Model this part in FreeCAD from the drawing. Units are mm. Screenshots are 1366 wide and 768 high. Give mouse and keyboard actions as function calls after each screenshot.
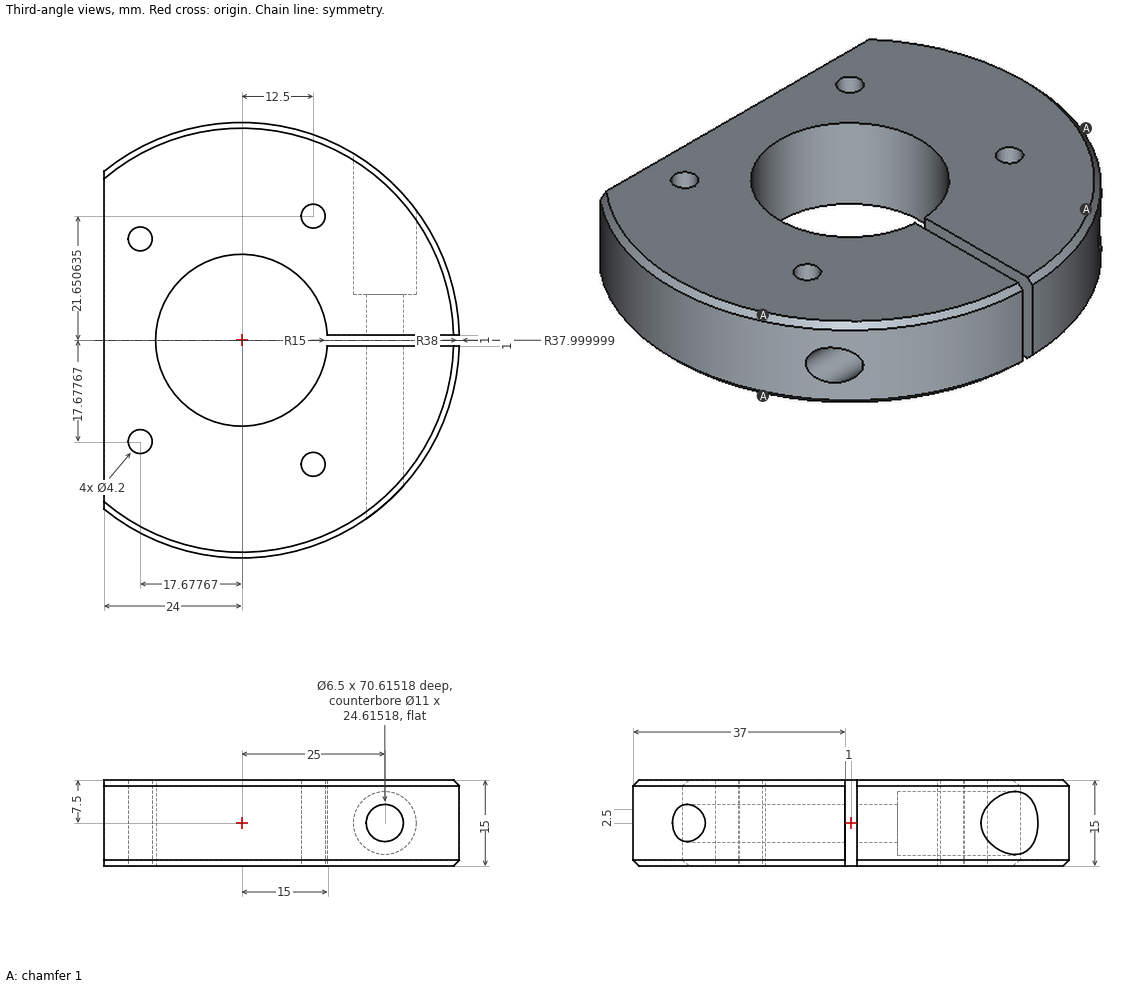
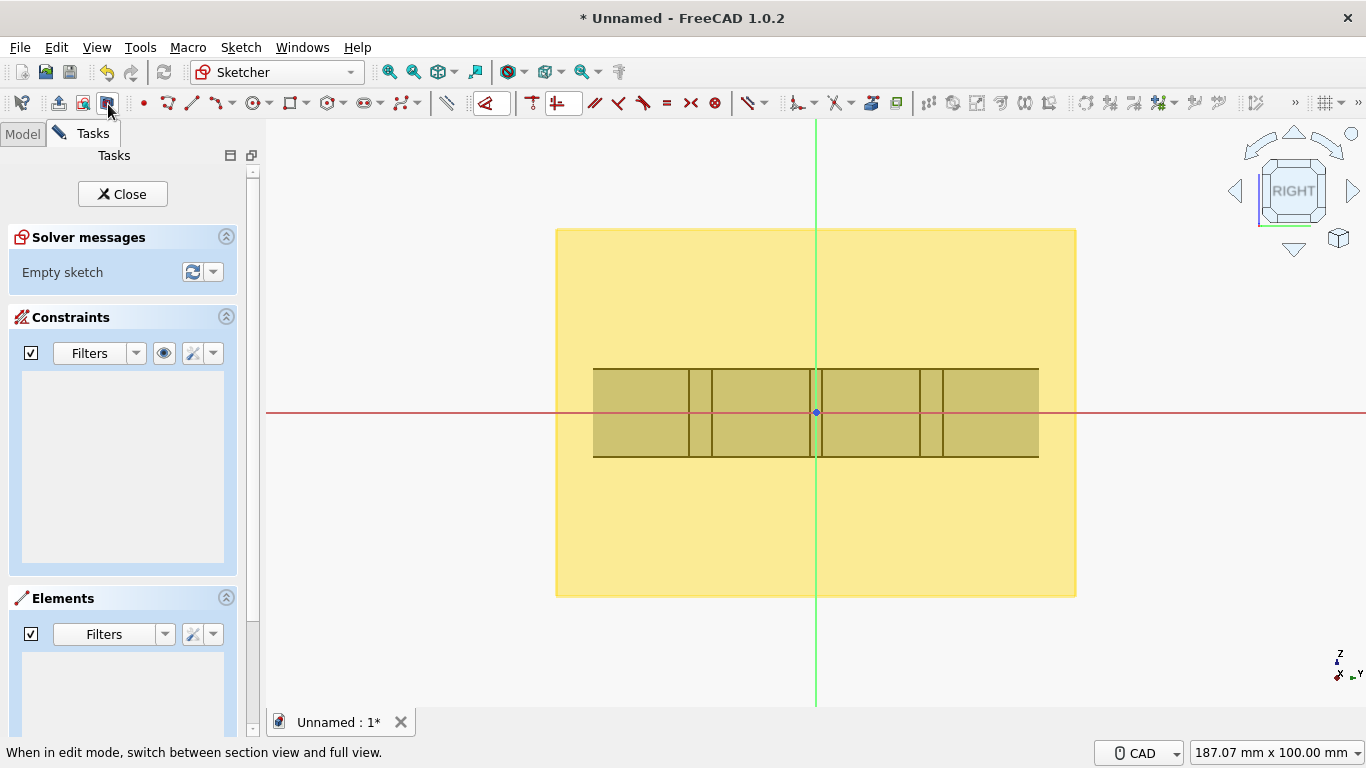
scroll(679, 401, up, 5)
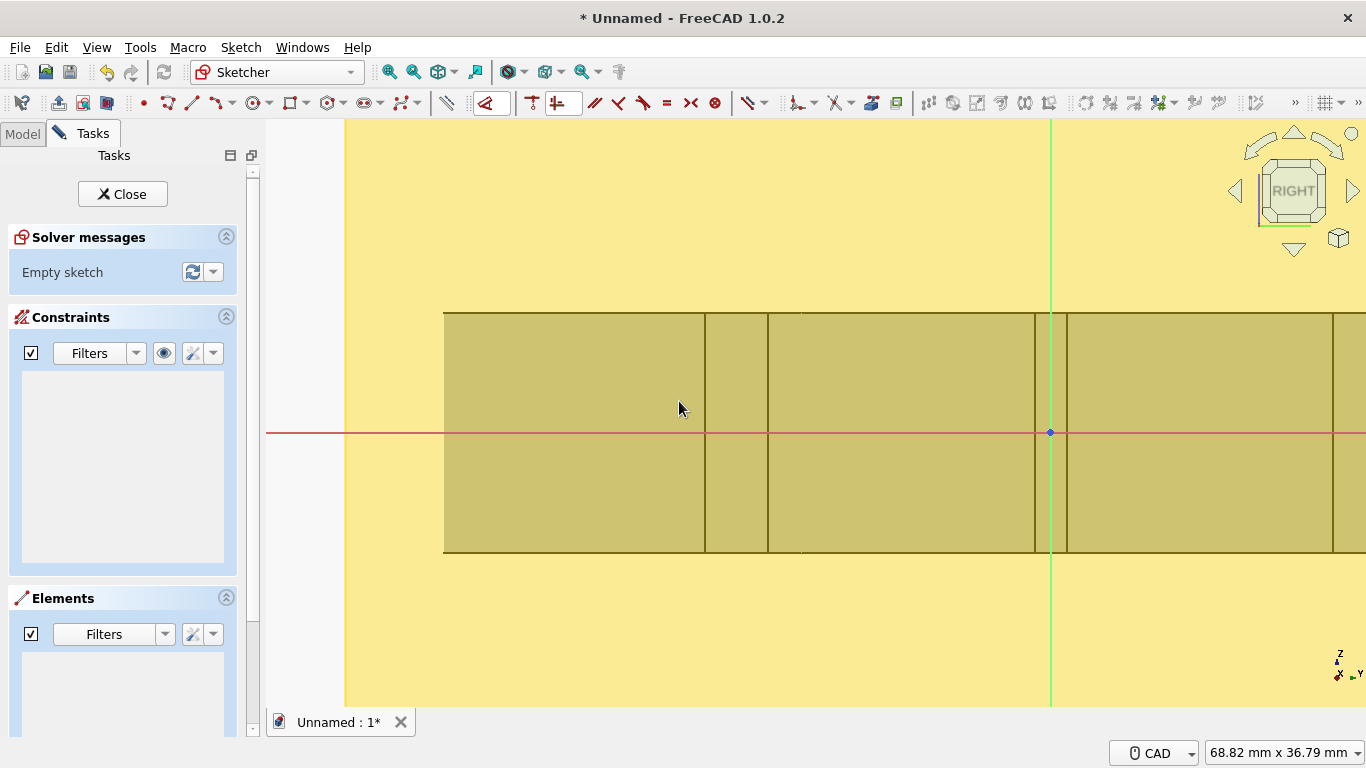
click(290, 104)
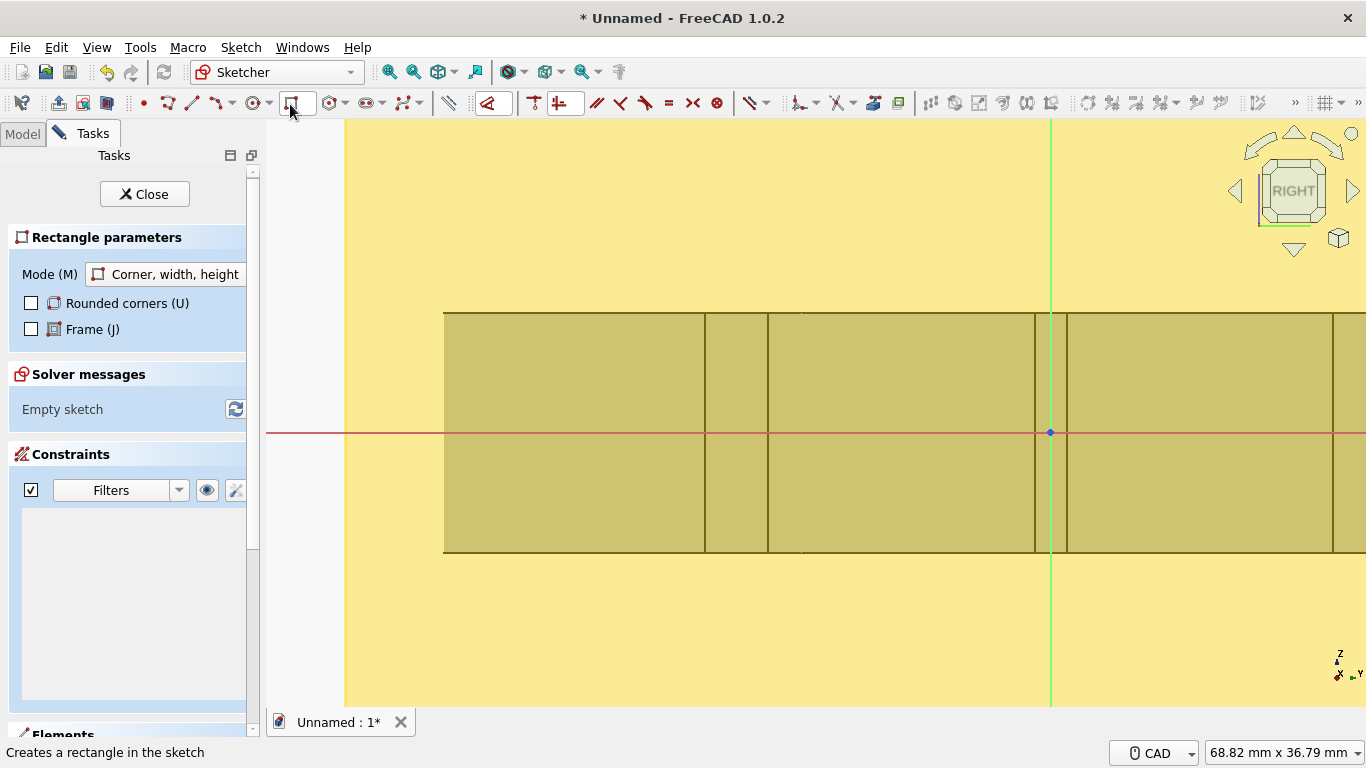
click(443, 393)
click(1035, 433)
key(Escape)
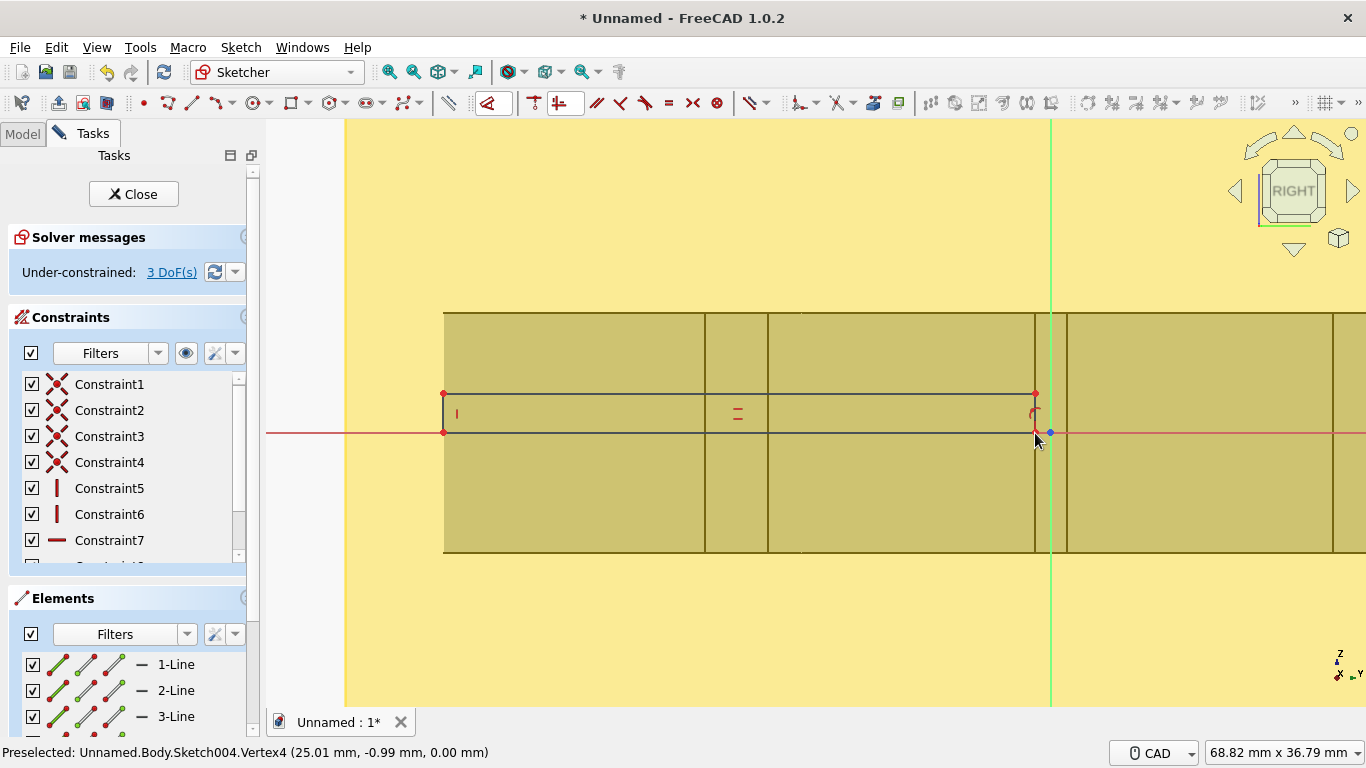
click(621, 433)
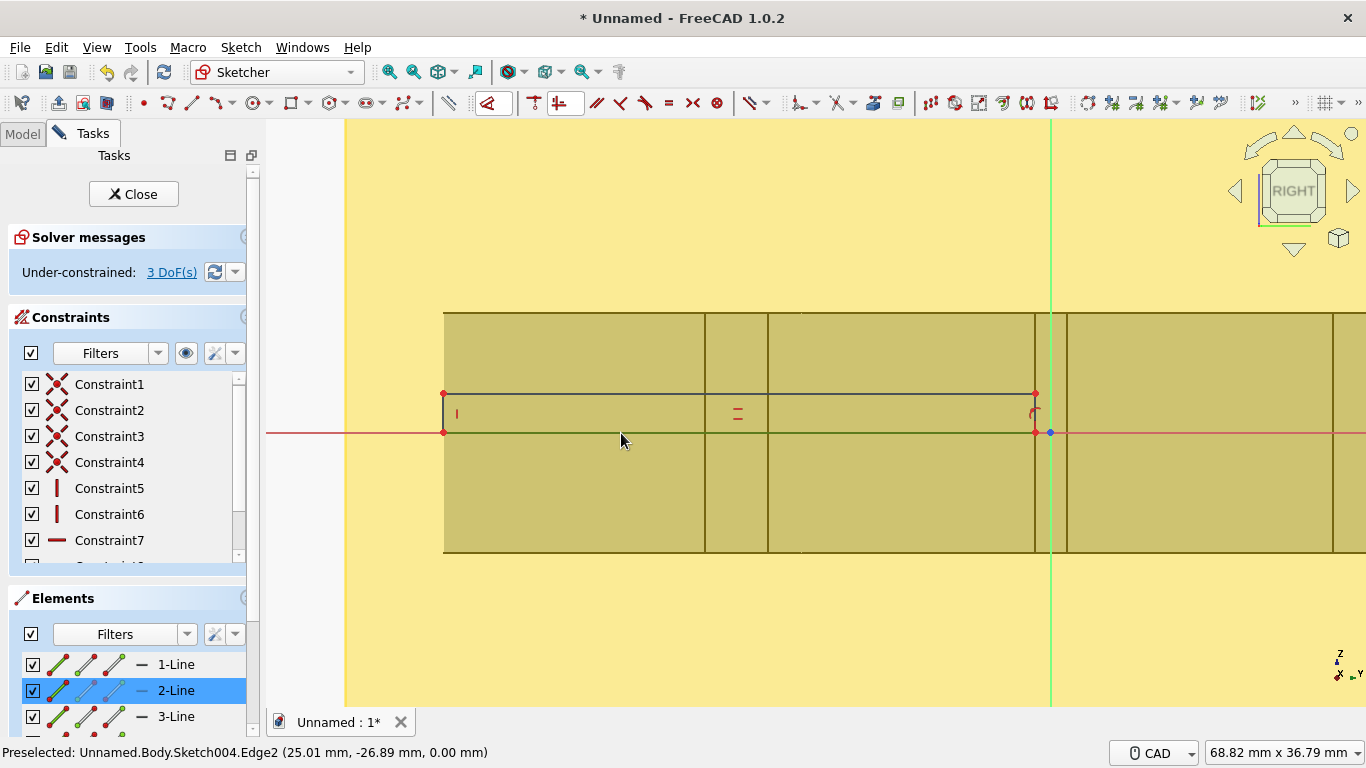
key(l)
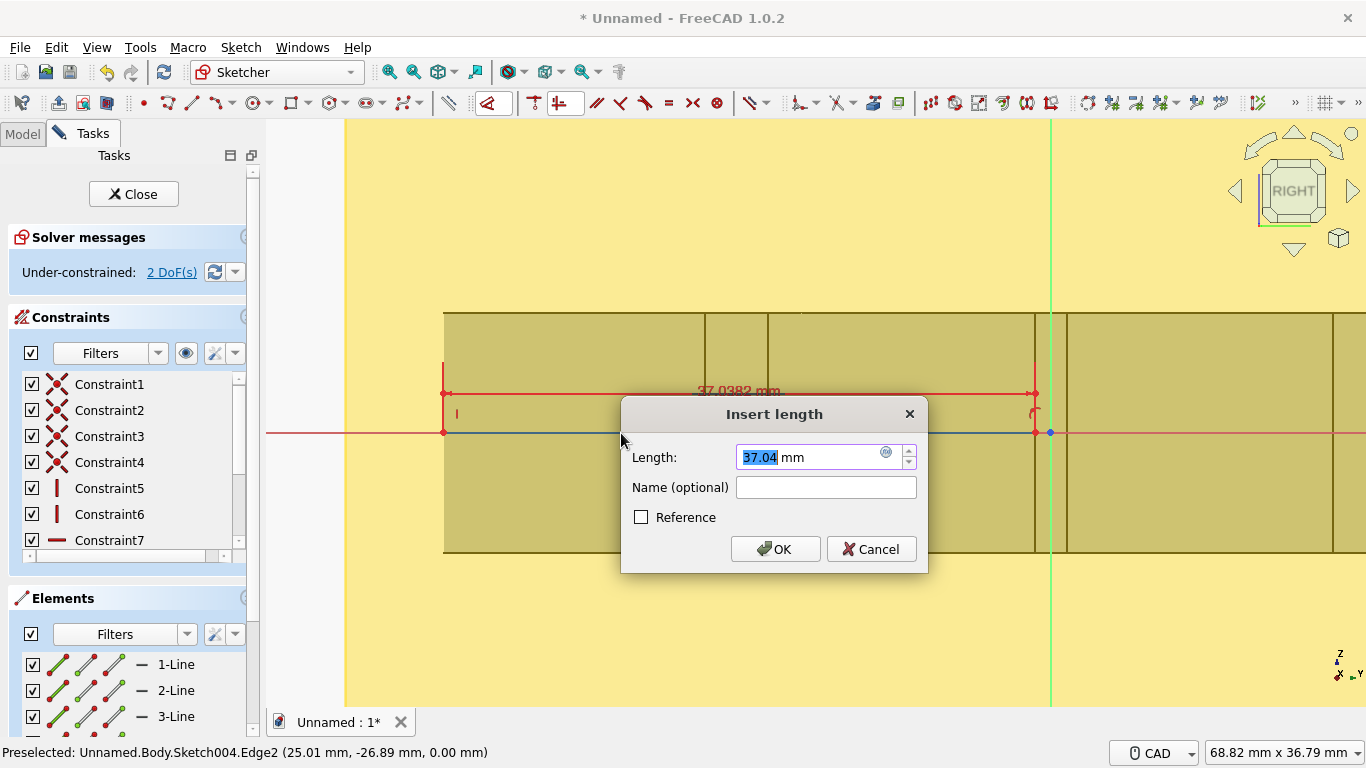
text(37)
key(Return)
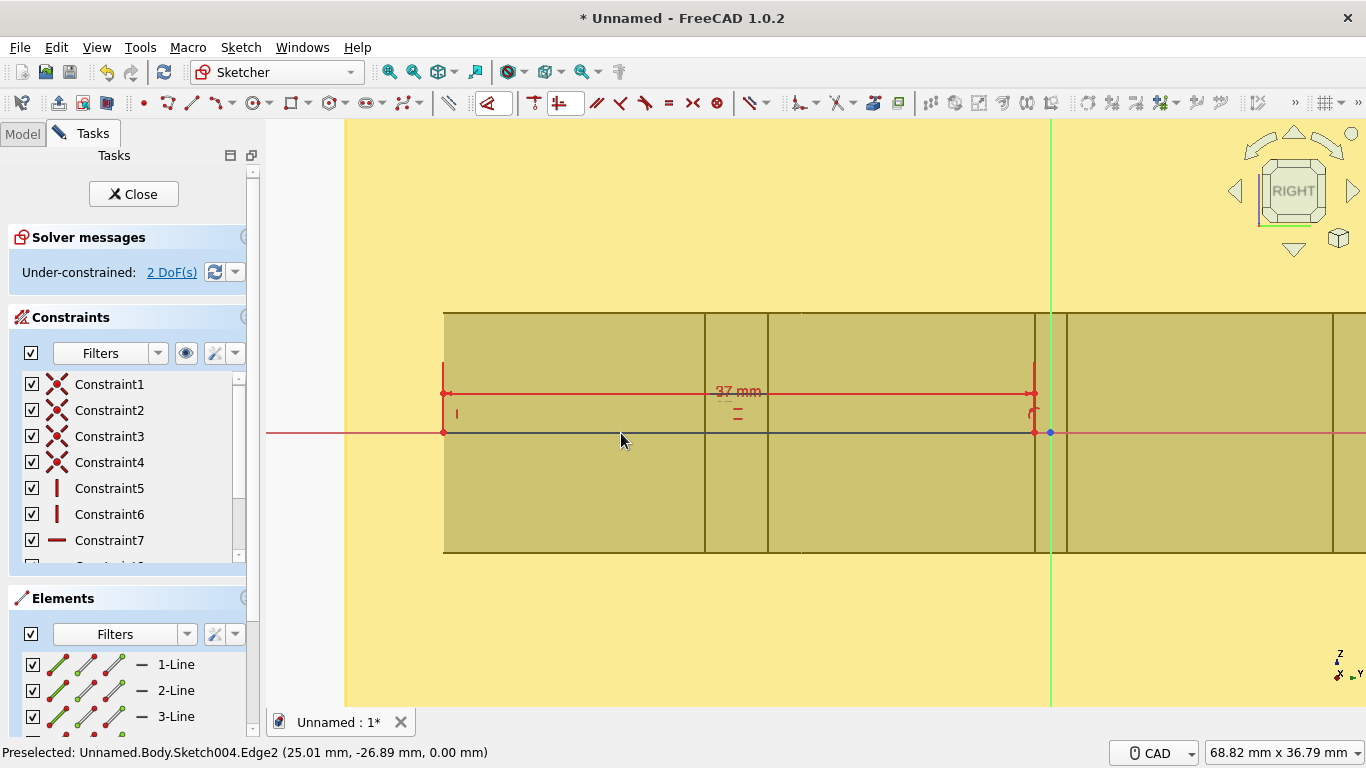
scroll(1034, 433, up, 5)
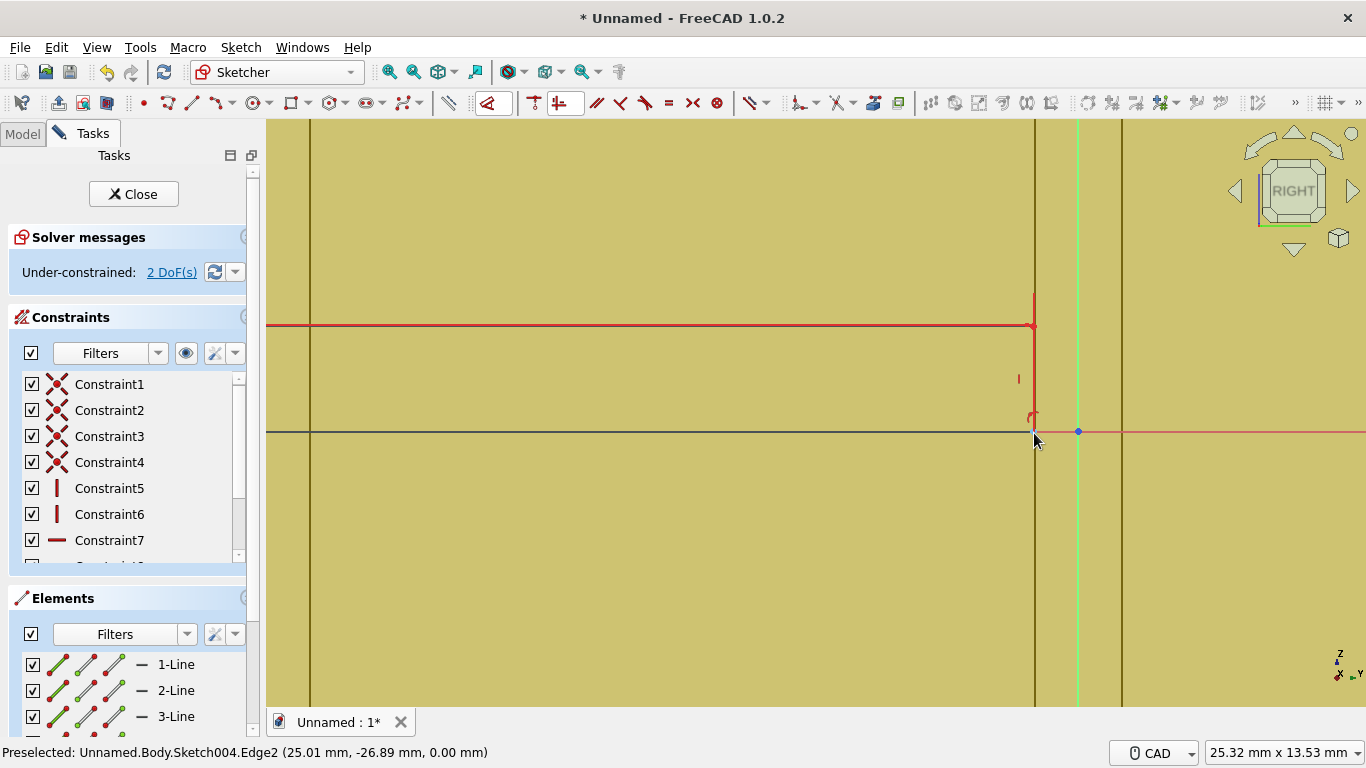
click(1034, 432)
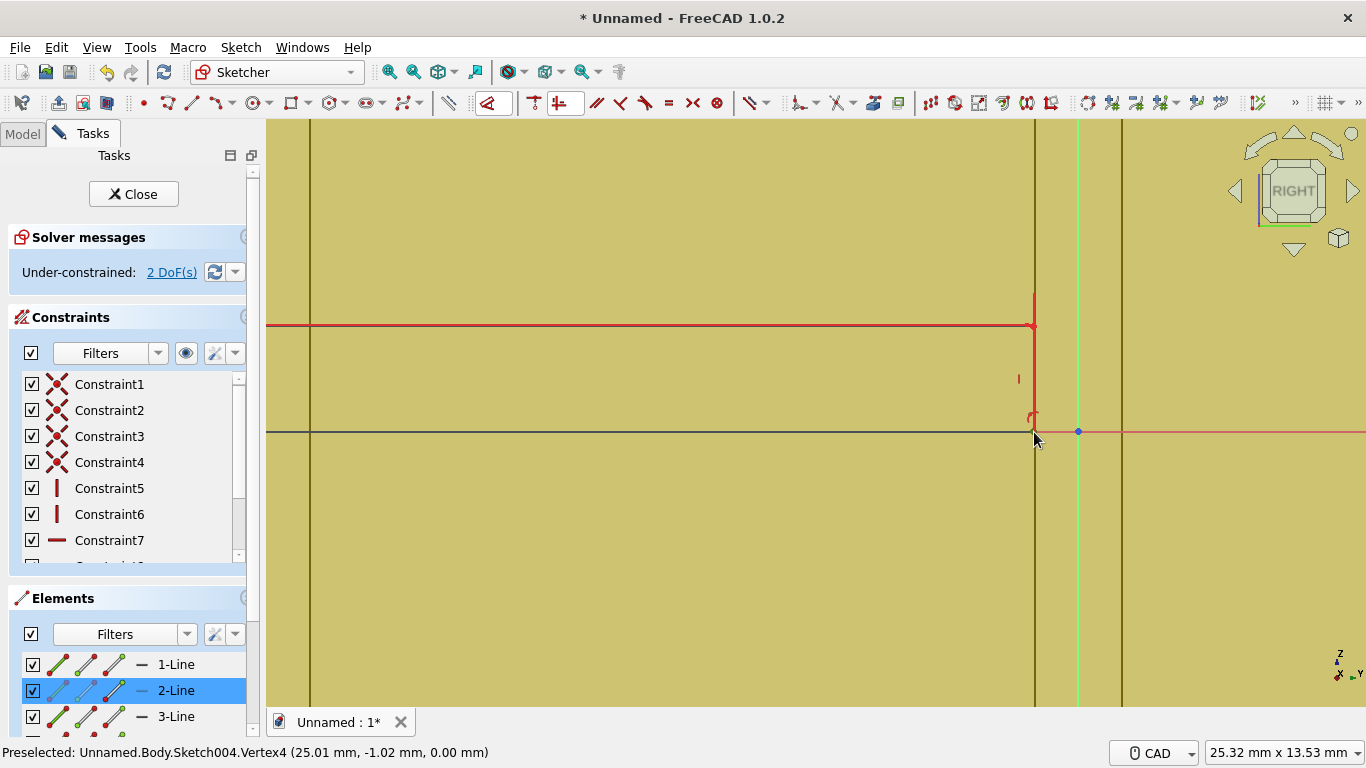
key(l)